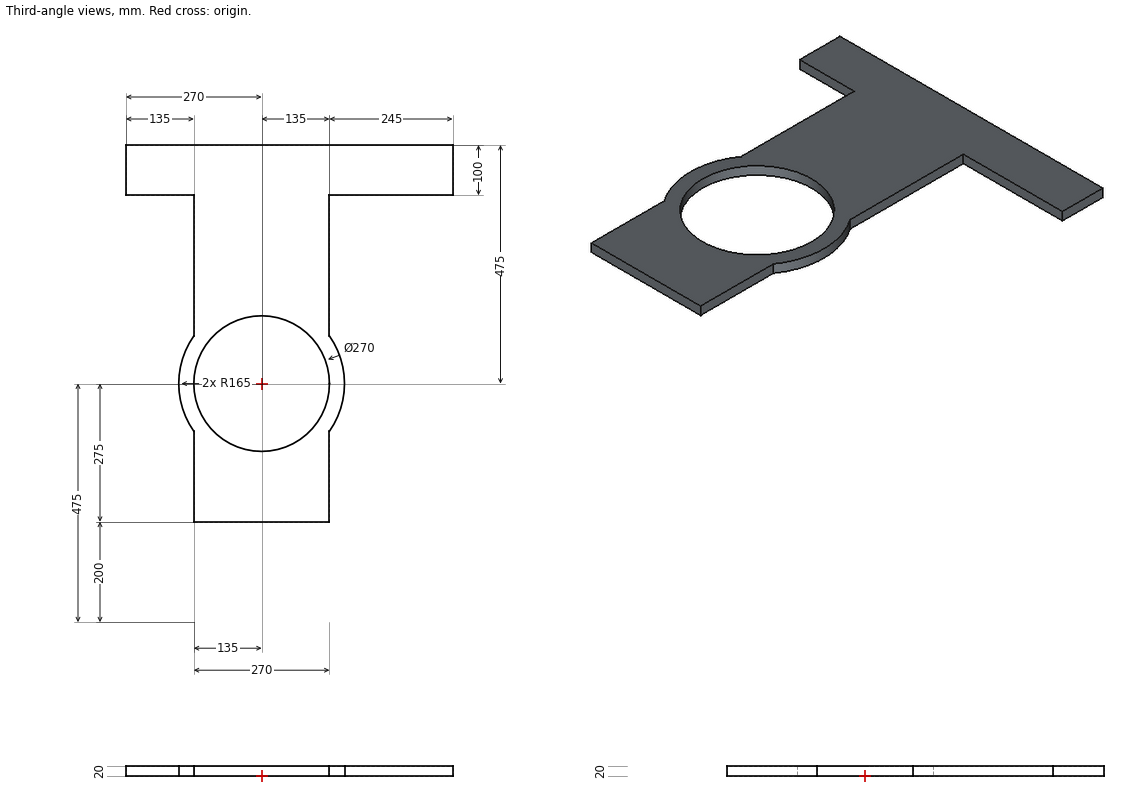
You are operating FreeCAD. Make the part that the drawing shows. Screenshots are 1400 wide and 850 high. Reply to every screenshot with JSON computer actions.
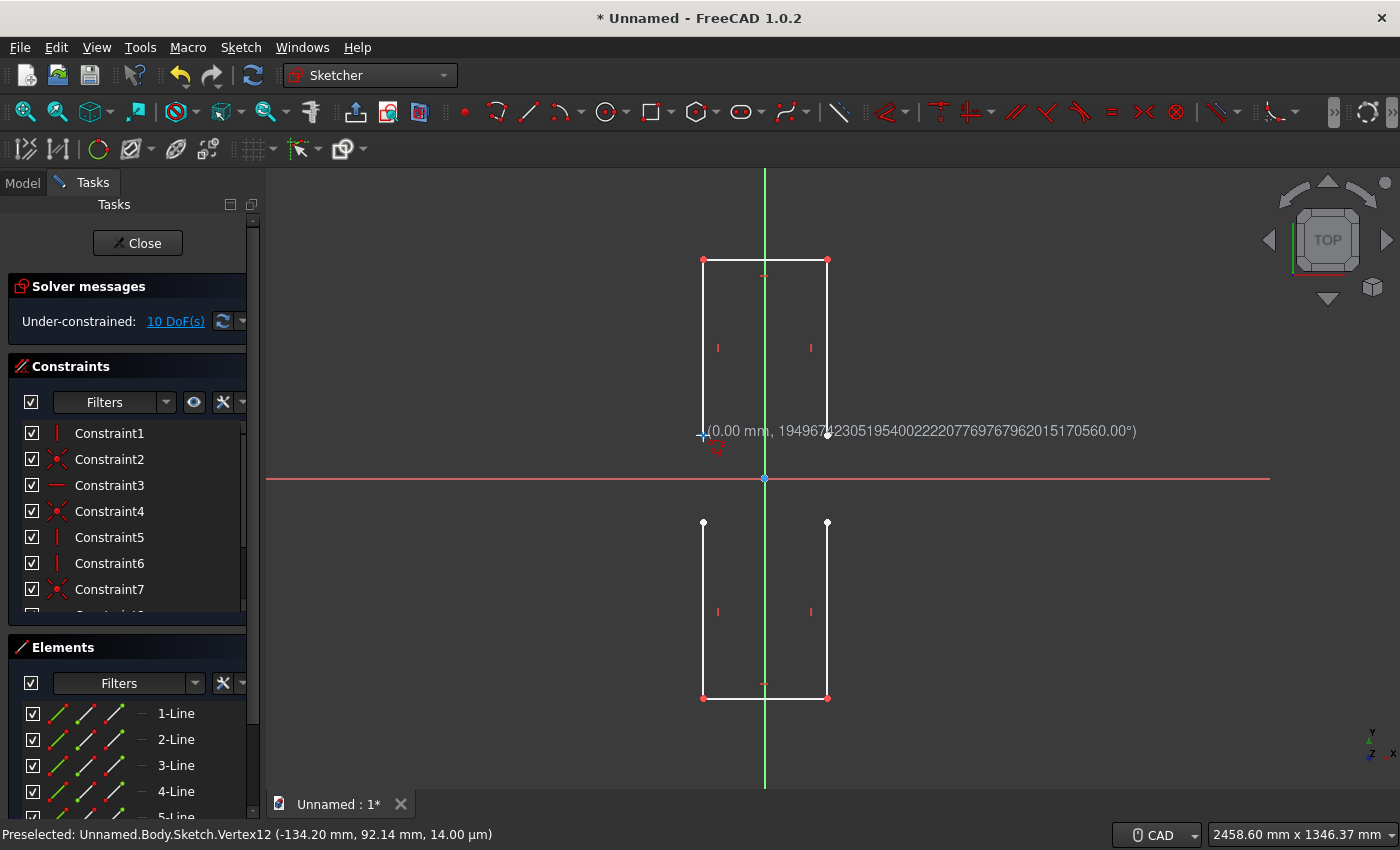
{"action": "key", "text": "g 3 a"}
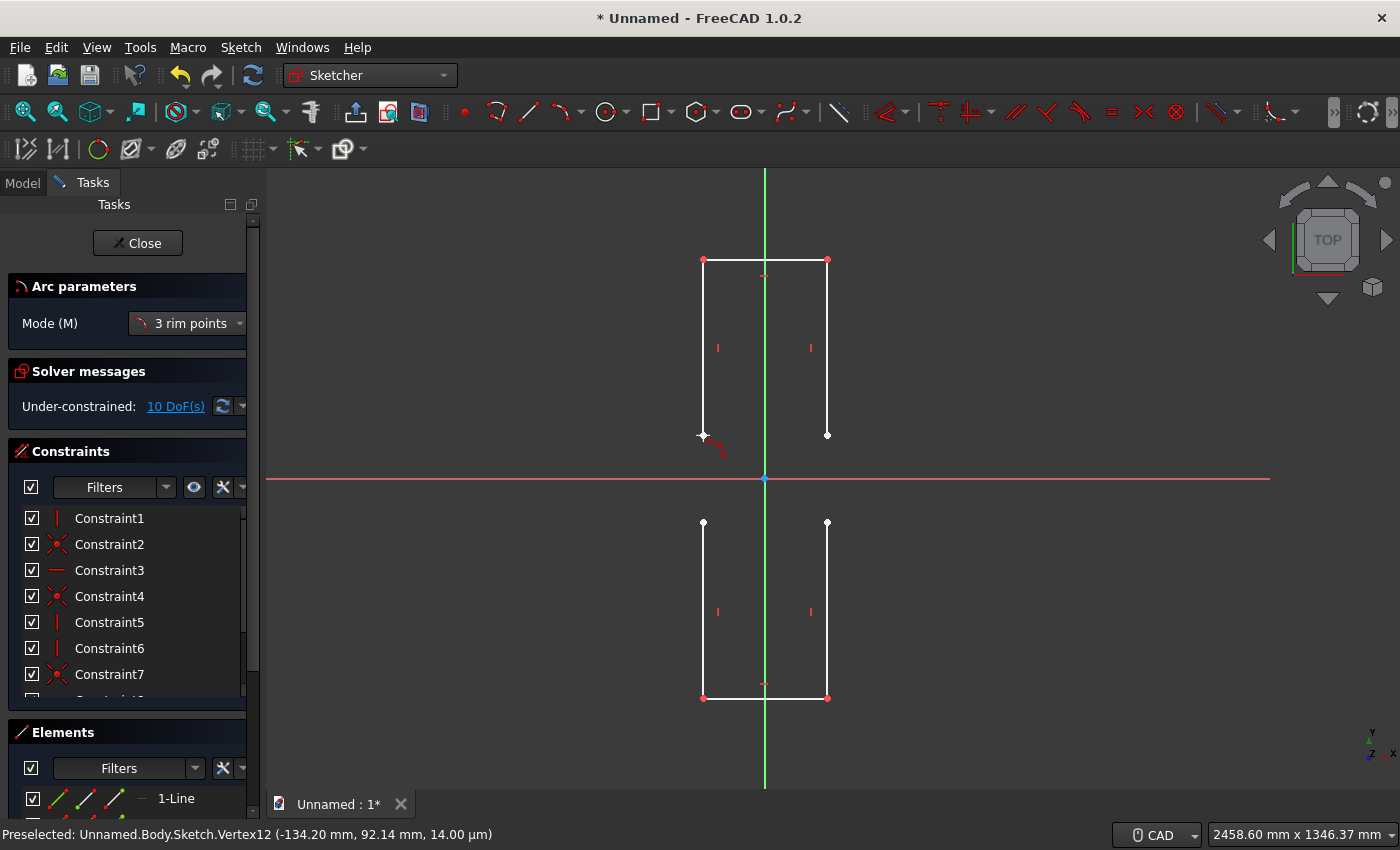
{"action": "left_click", "coordinate": [827, 523]}
{"action": "left_click", "coordinate": [827, 436]}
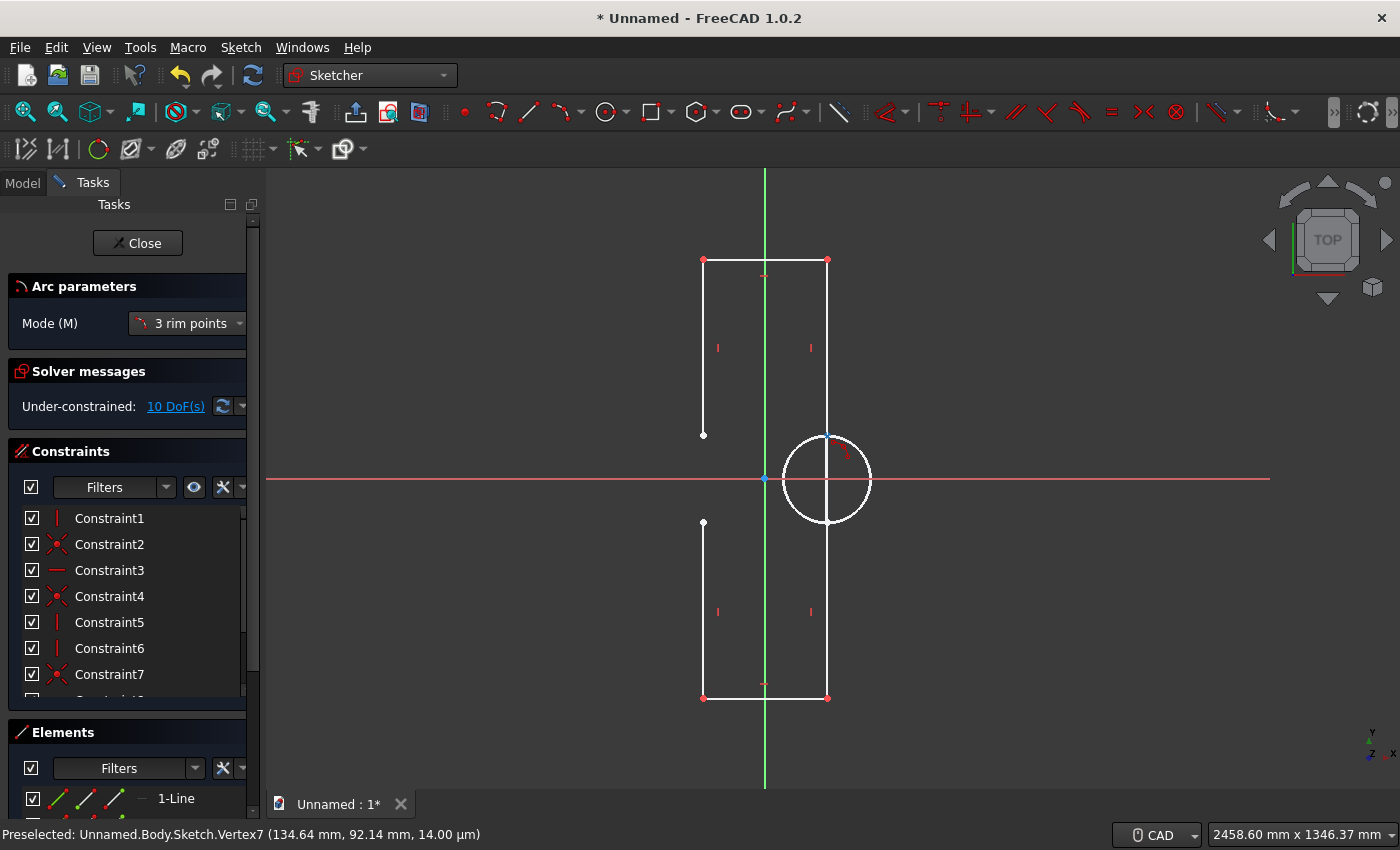
{"action": "scroll", "coordinate": [839, 497], "scroll_direction": "up", "scroll_amount": 2}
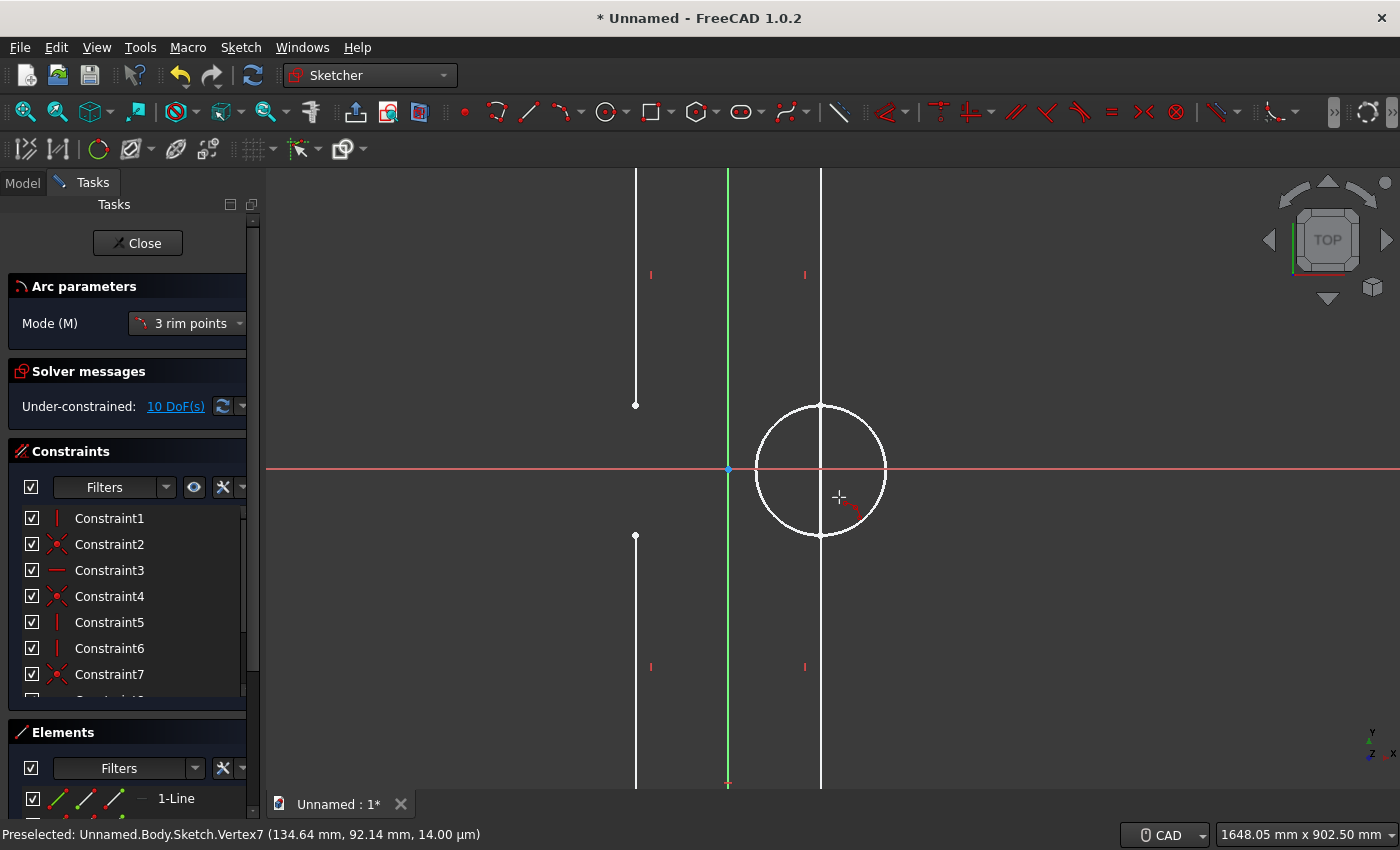
{"action": "left_click", "coordinate": [838, 497]}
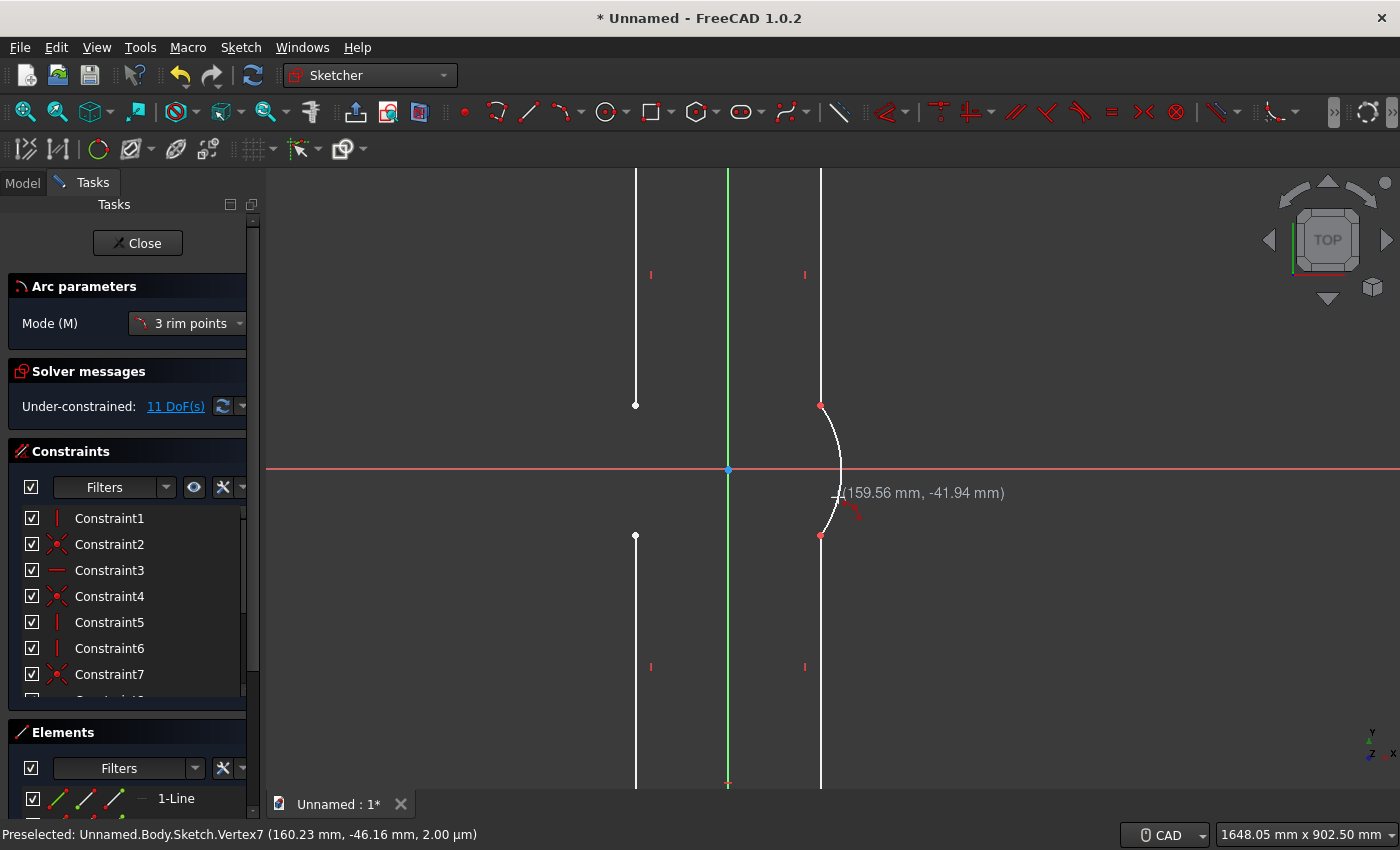
{"action": "left_click", "coordinate": [636, 406]}
{"action": "left_click", "coordinate": [636, 536]}
{"action": "left_click", "coordinate": [618, 497]}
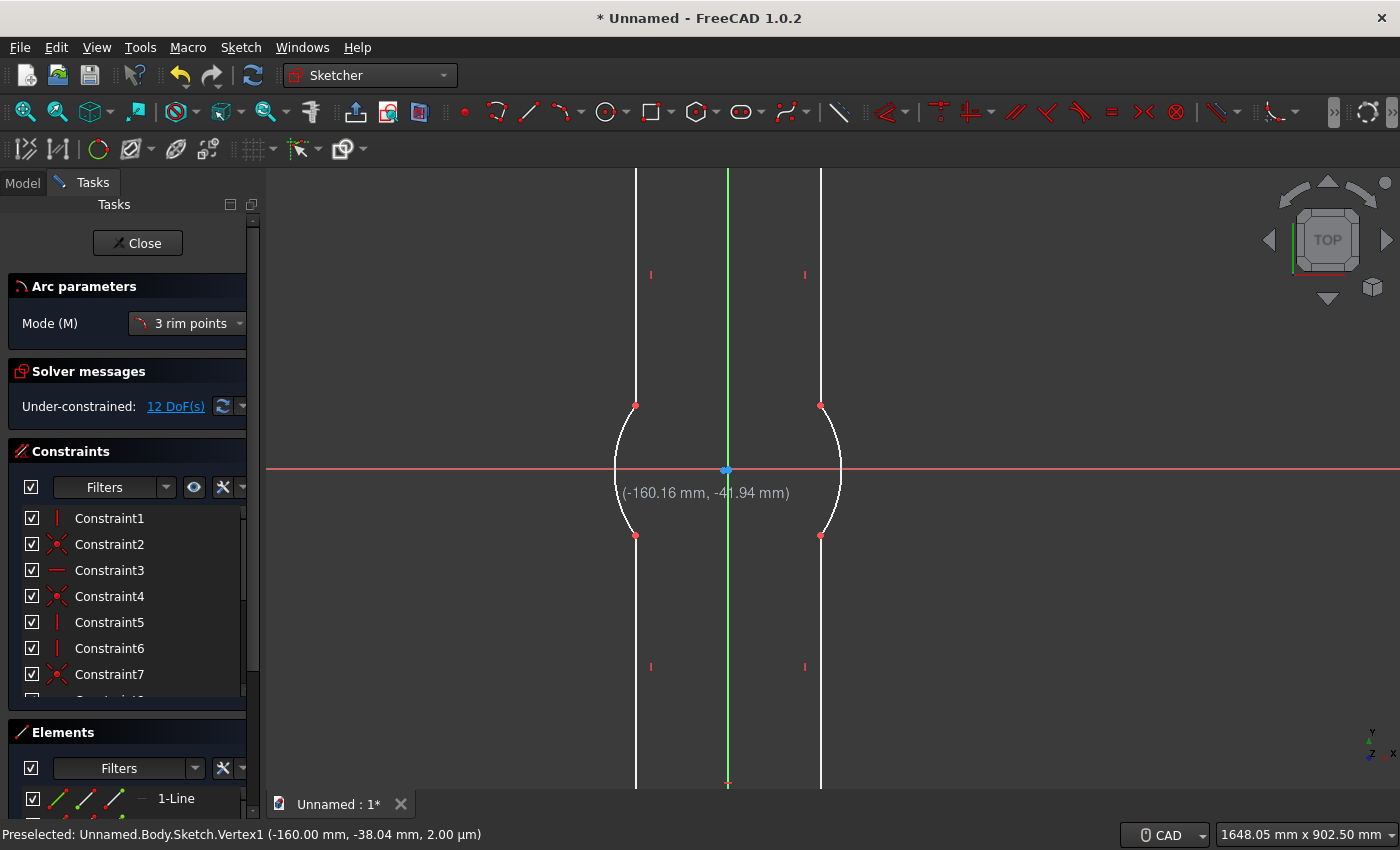
{"action": "left_click", "coordinate": [606, 112]}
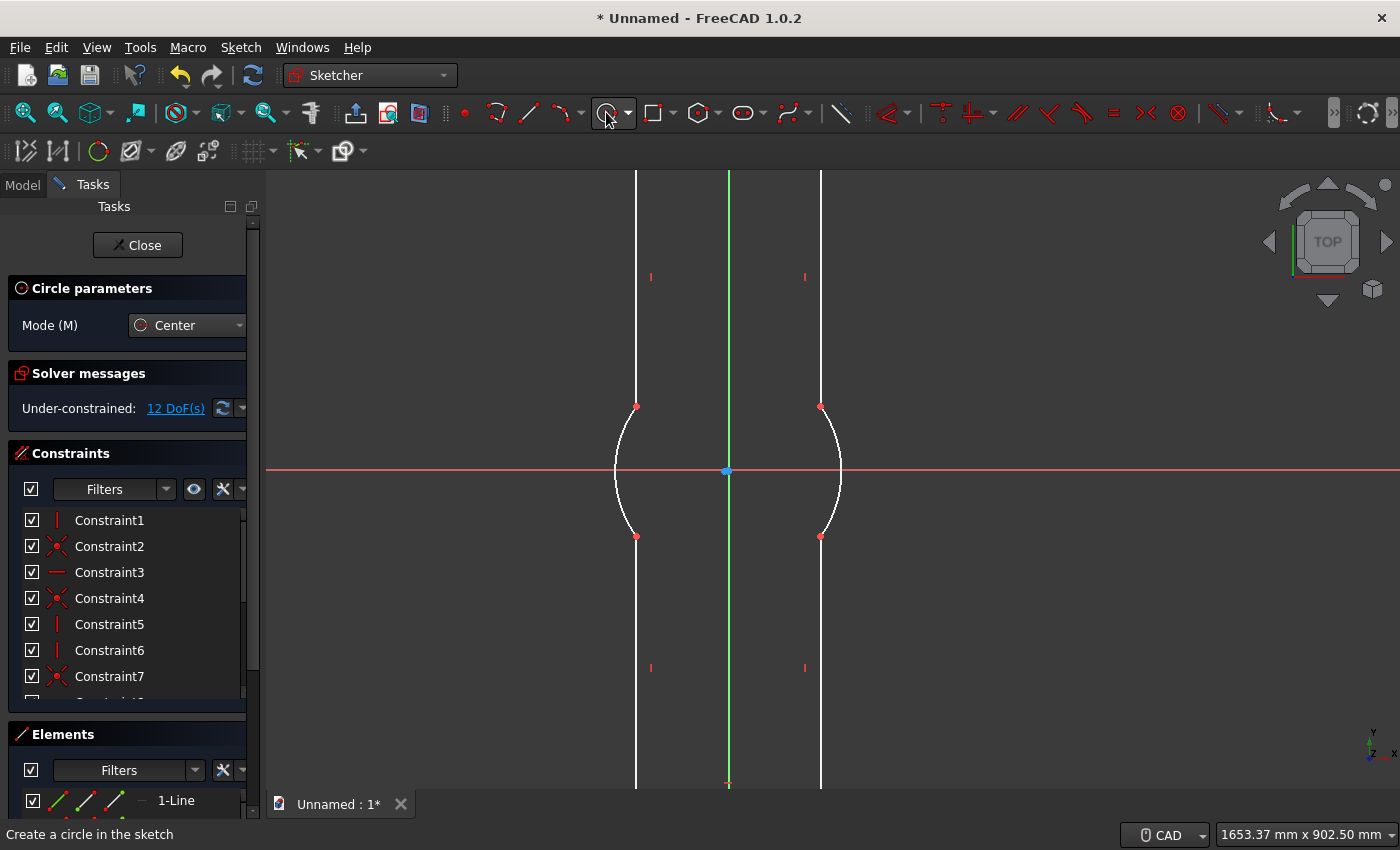
{"action": "left_click", "coordinate": [729, 470]}
{"action": "left_click", "coordinate": [794, 405]}
{"action": "key", "text": "Escape"}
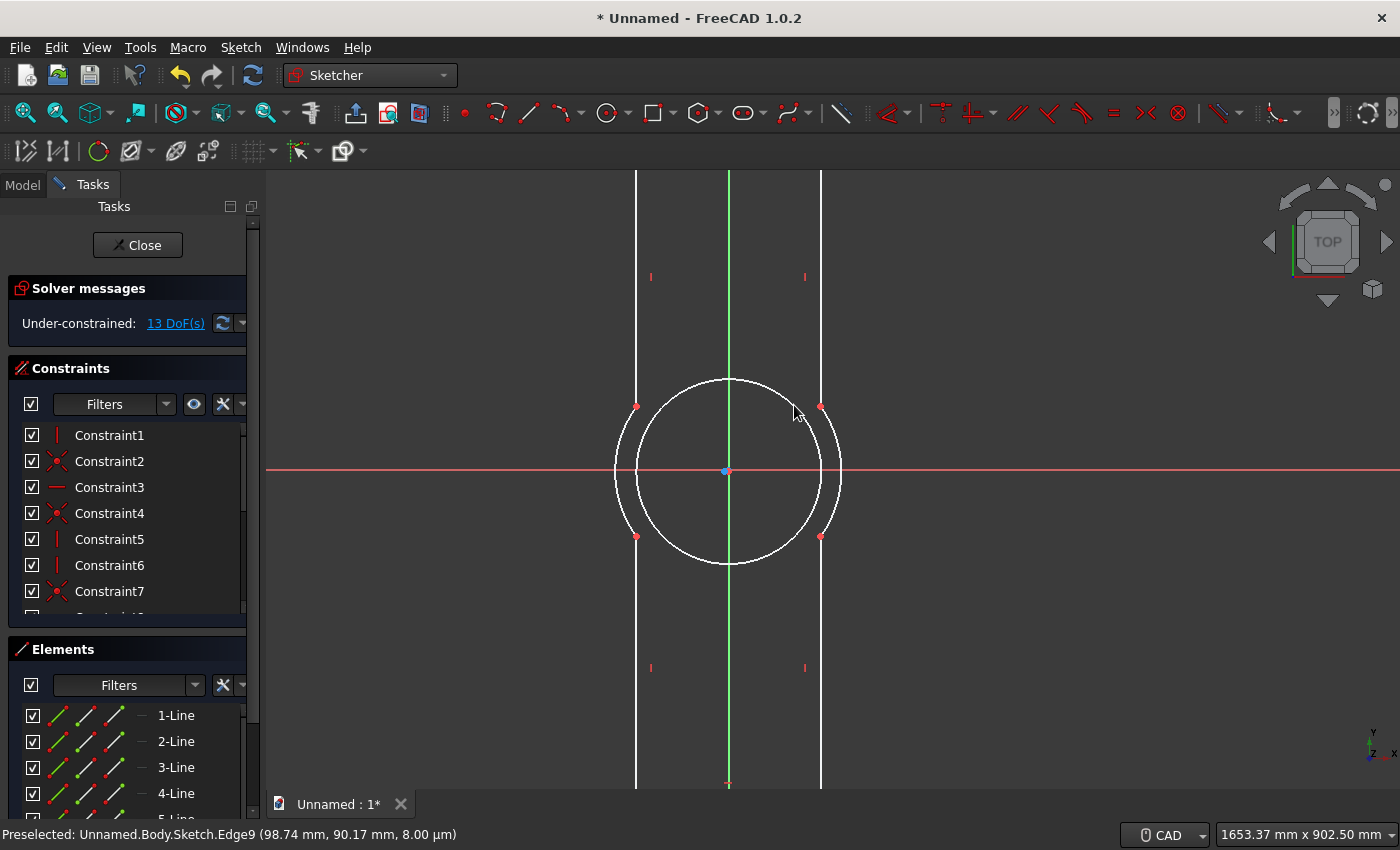
{"action": "left_click", "coordinate": [794, 406]}